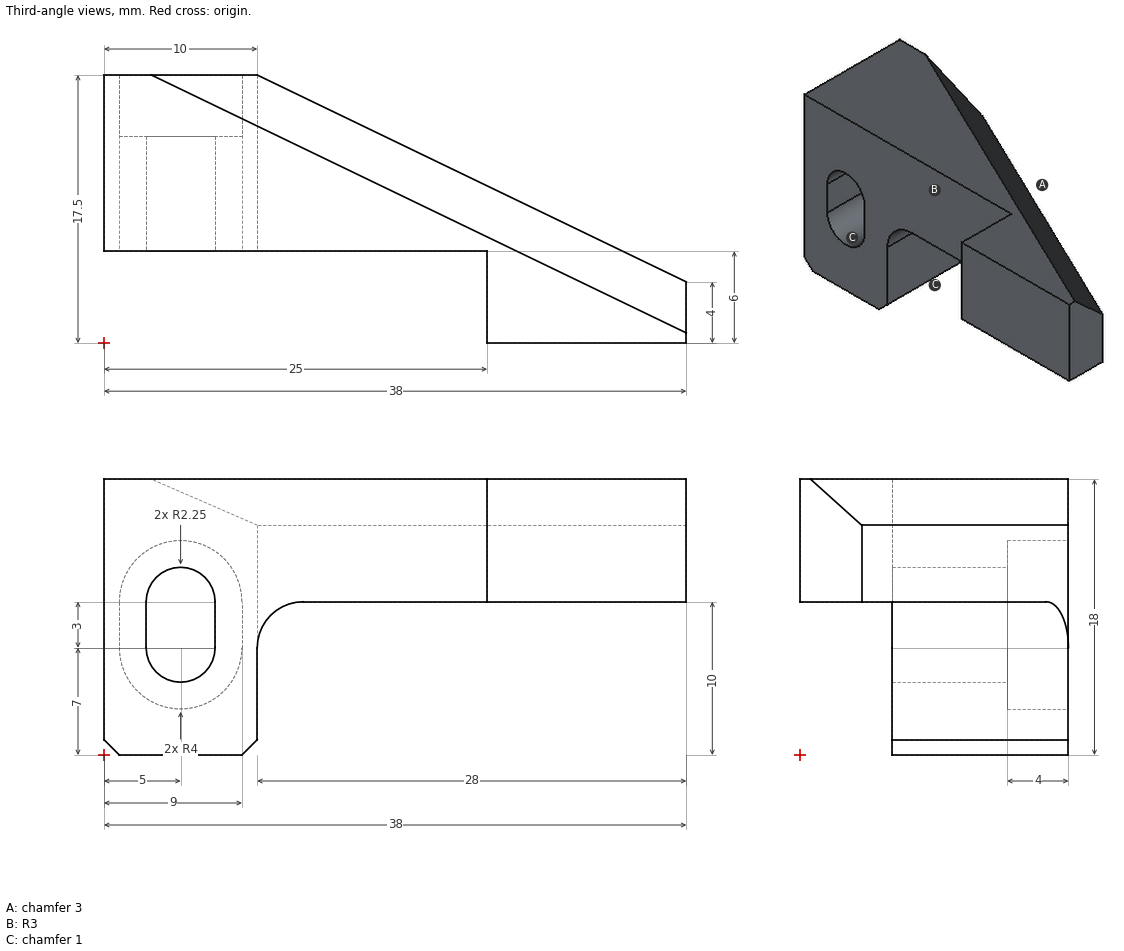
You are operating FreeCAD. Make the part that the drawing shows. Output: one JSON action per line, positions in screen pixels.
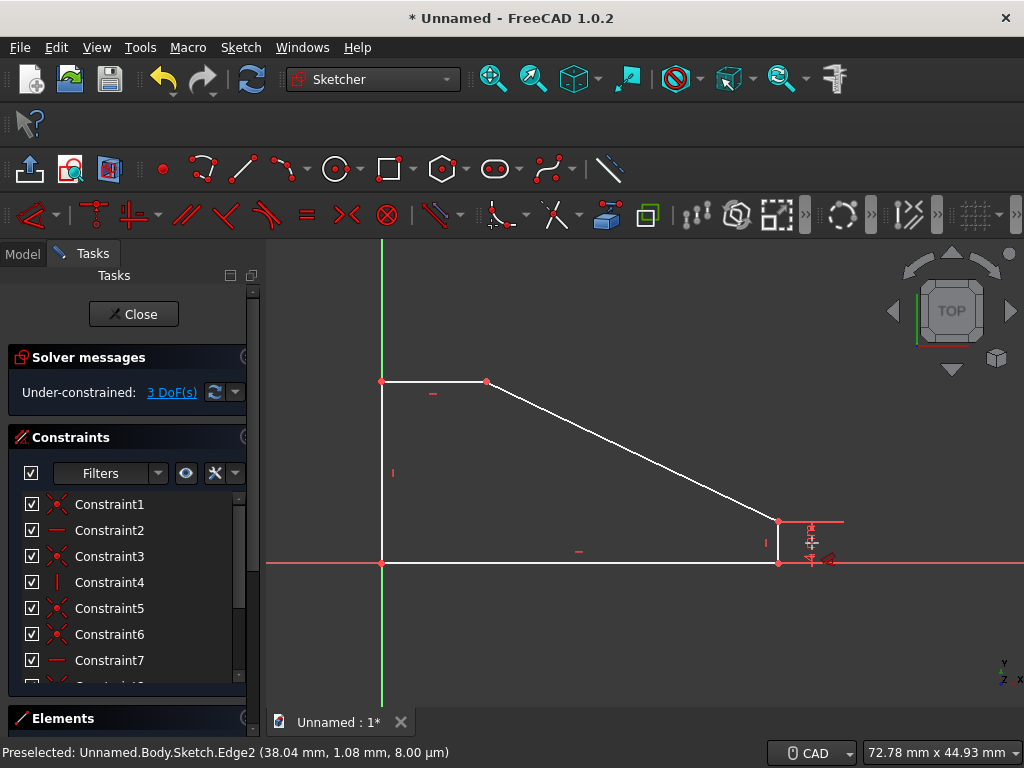
{"action": "left_click", "coordinate": [501, 563]}
{"action": "left_click", "coordinate": [580, 597]}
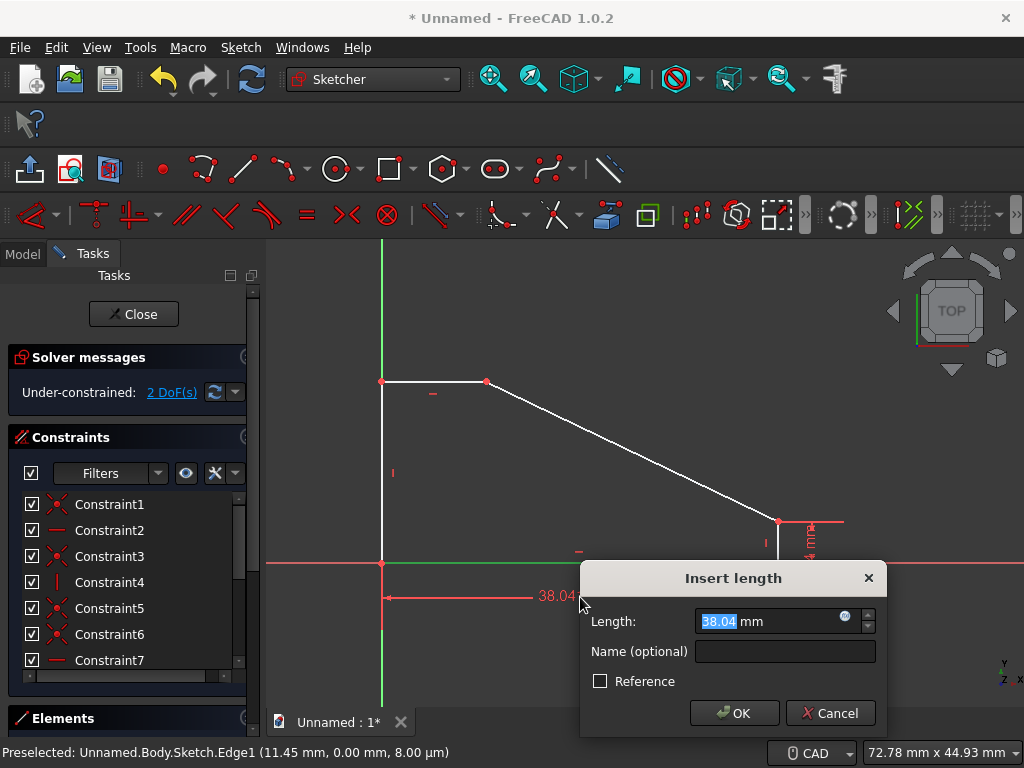
{"action": "type", "text": "38"}
{"action": "key", "text": "Return"}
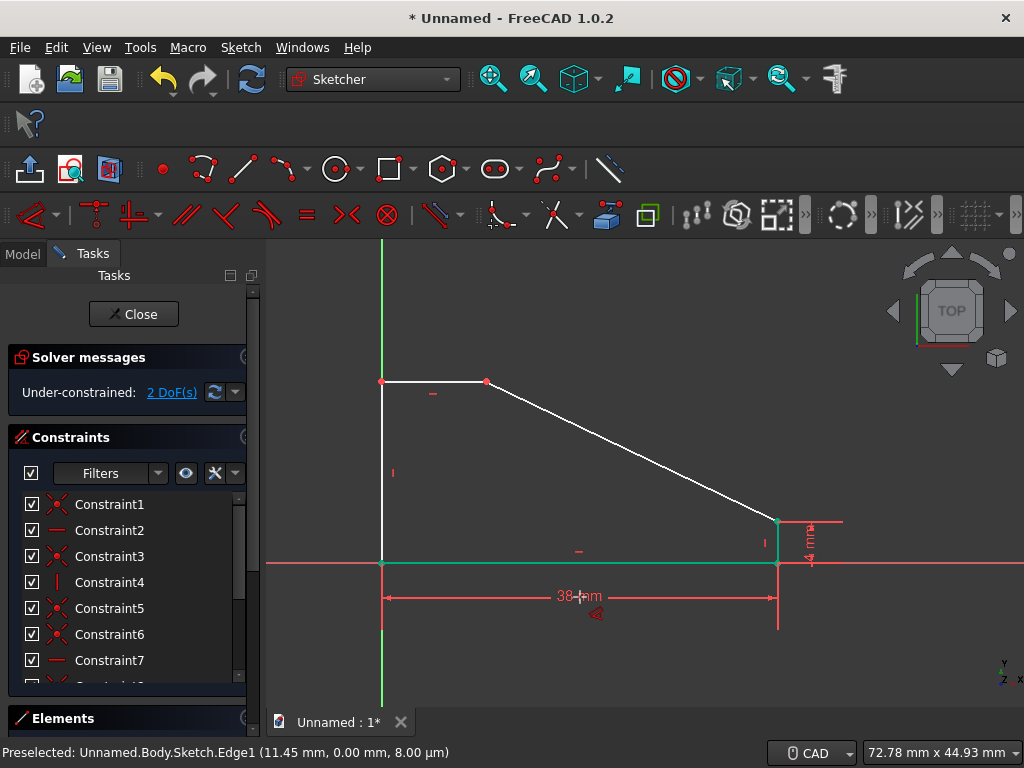
{"action": "left_click", "coordinate": [455, 382]}
{"action": "left_click", "coordinate": [434, 348]}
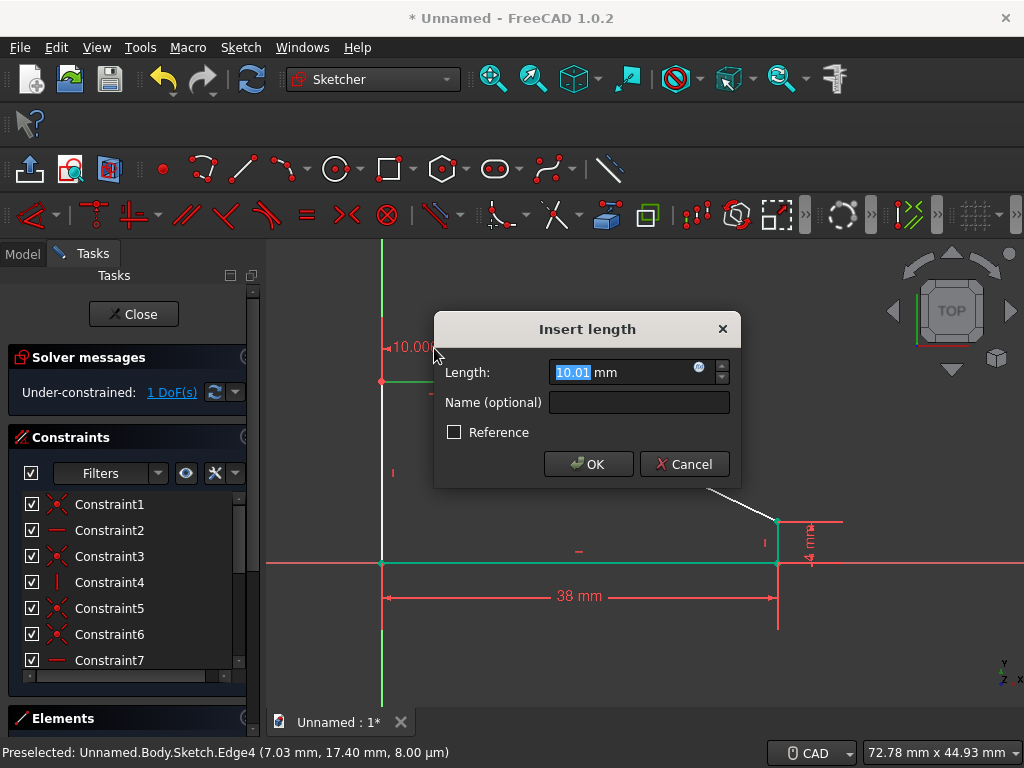
{"action": "type", "text": "10"}
{"action": "key", "text": "Return"}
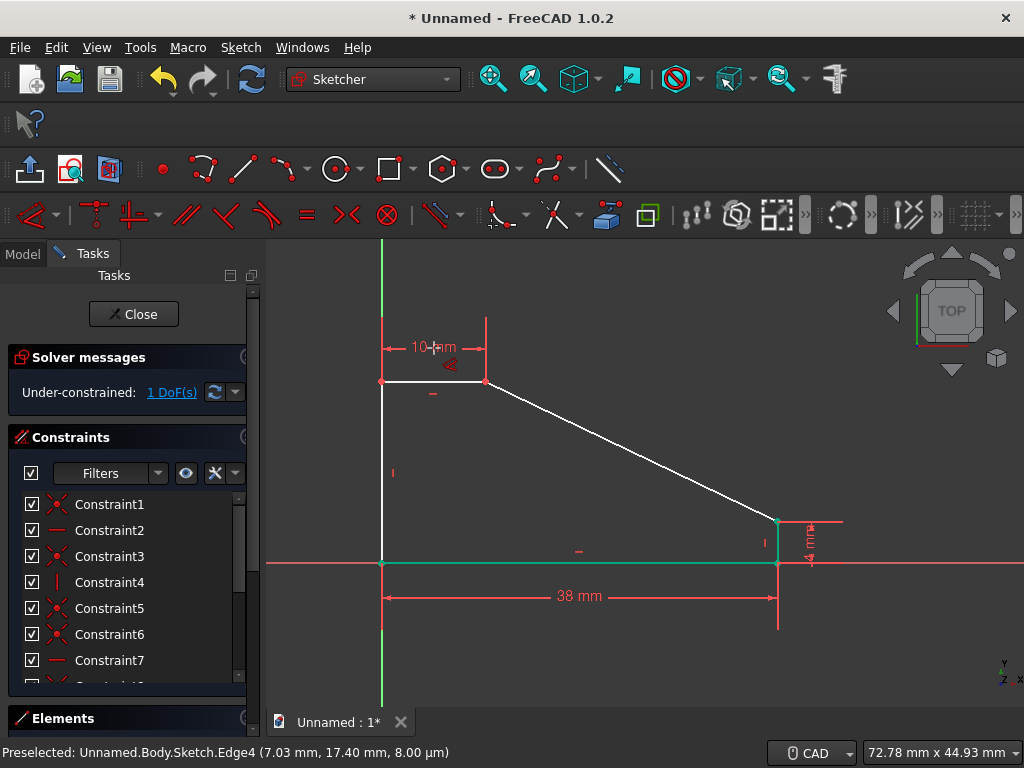
{"action": "left_click", "coordinate": [382, 436]}
{"action": "left_click", "coordinate": [348, 473]}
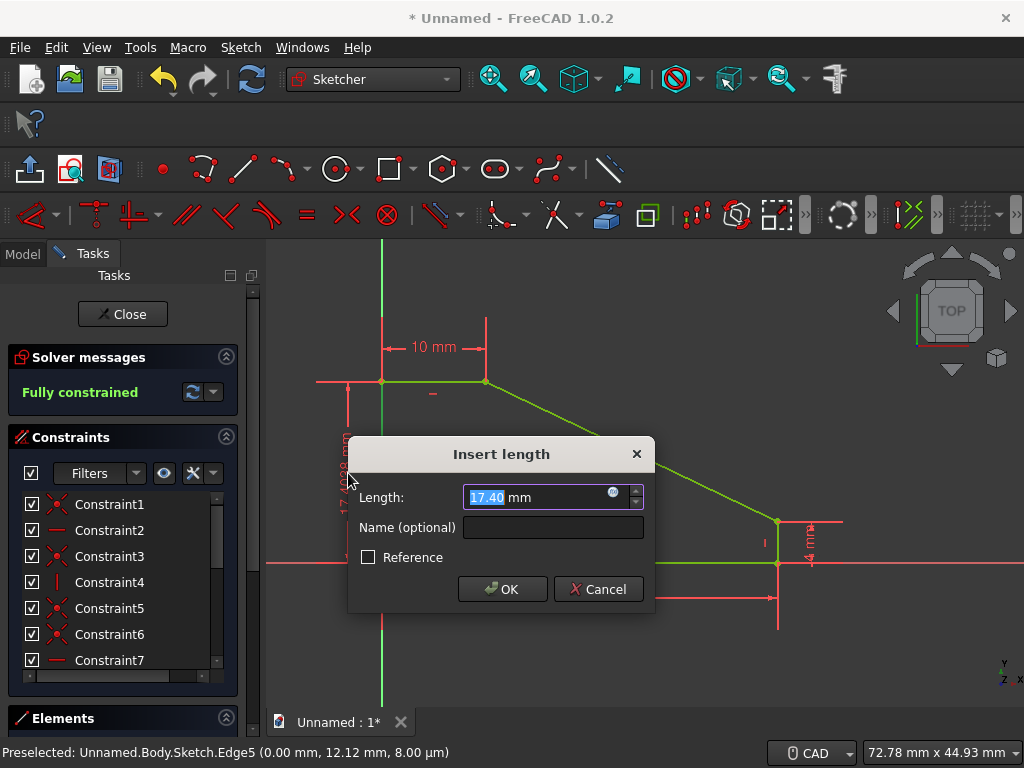
{"action": "type", "text": "17.5"}
{"action": "key", "text": "Return"}
{"action": "key", "text": "Escape"}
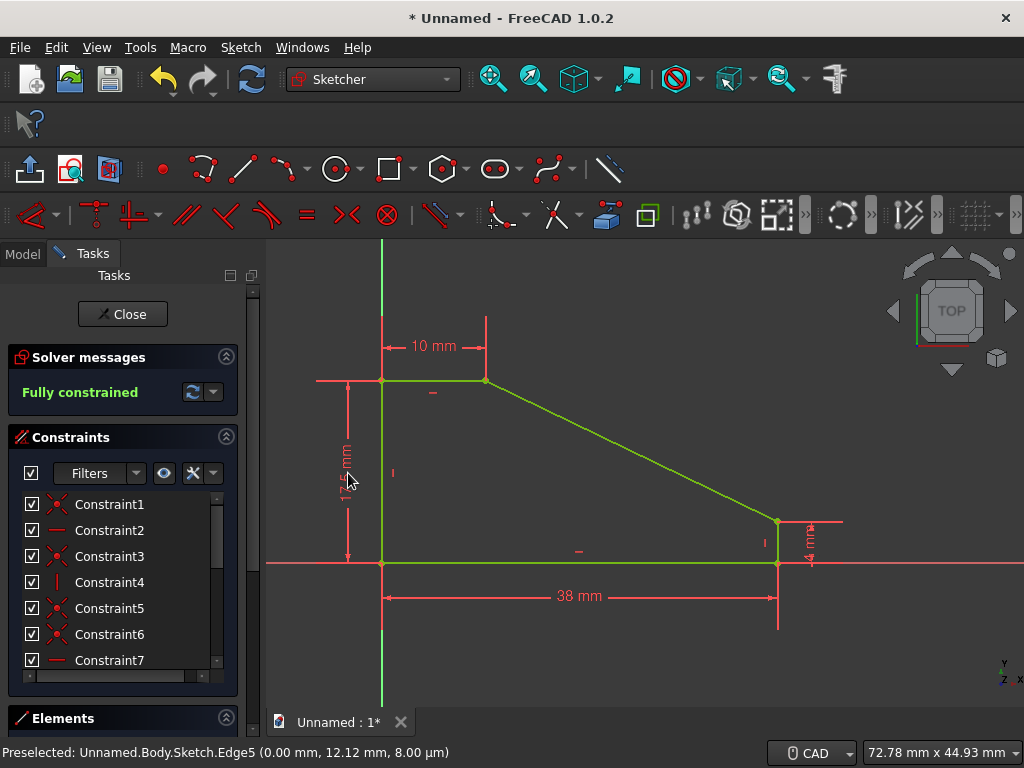
{"action": "left_click", "coordinate": [123, 314]}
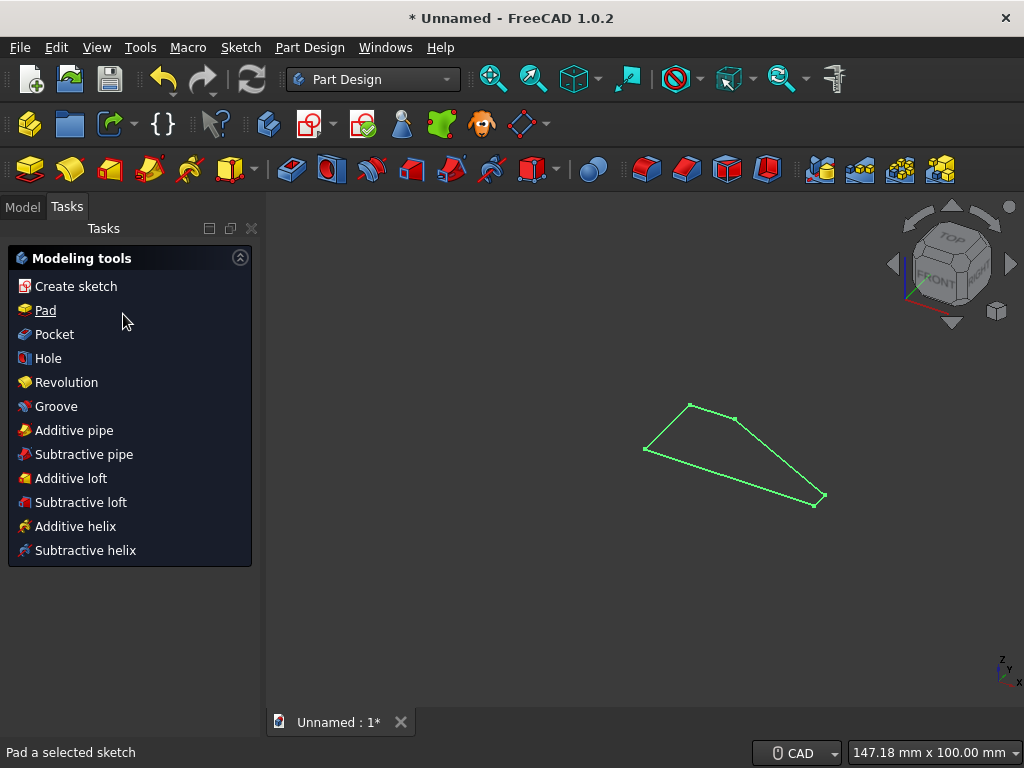
{"action": "left_click", "coordinate": [30, 170]}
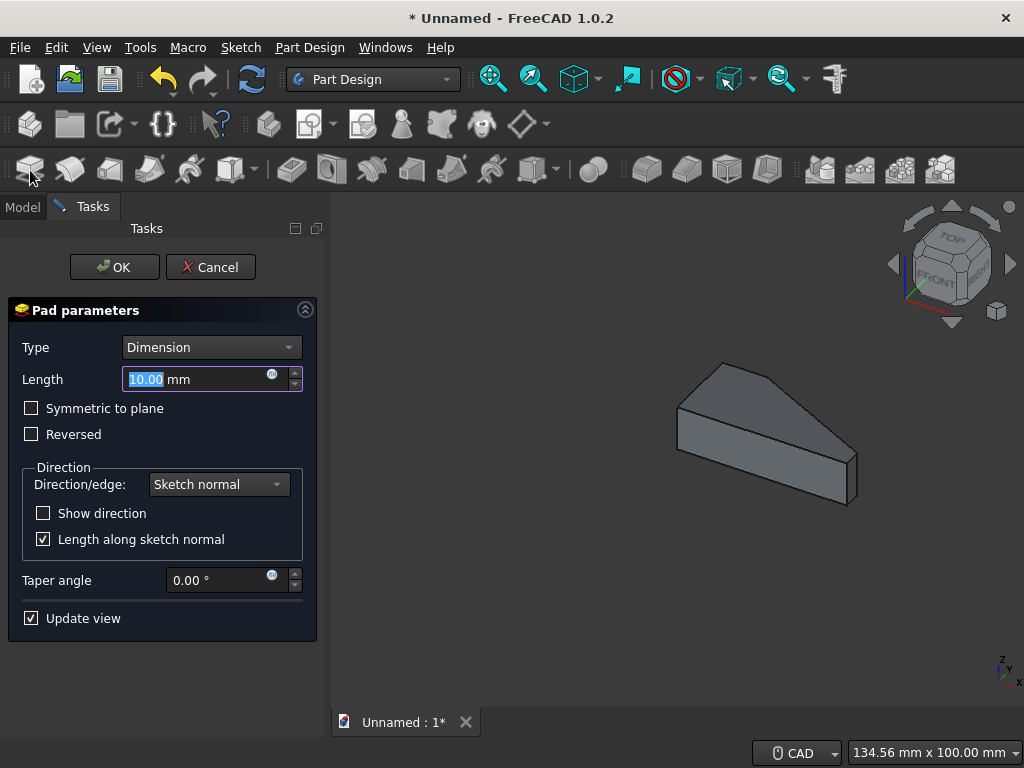
{"action": "type", "text": "18"}
{"action": "key", "text": "Tab"}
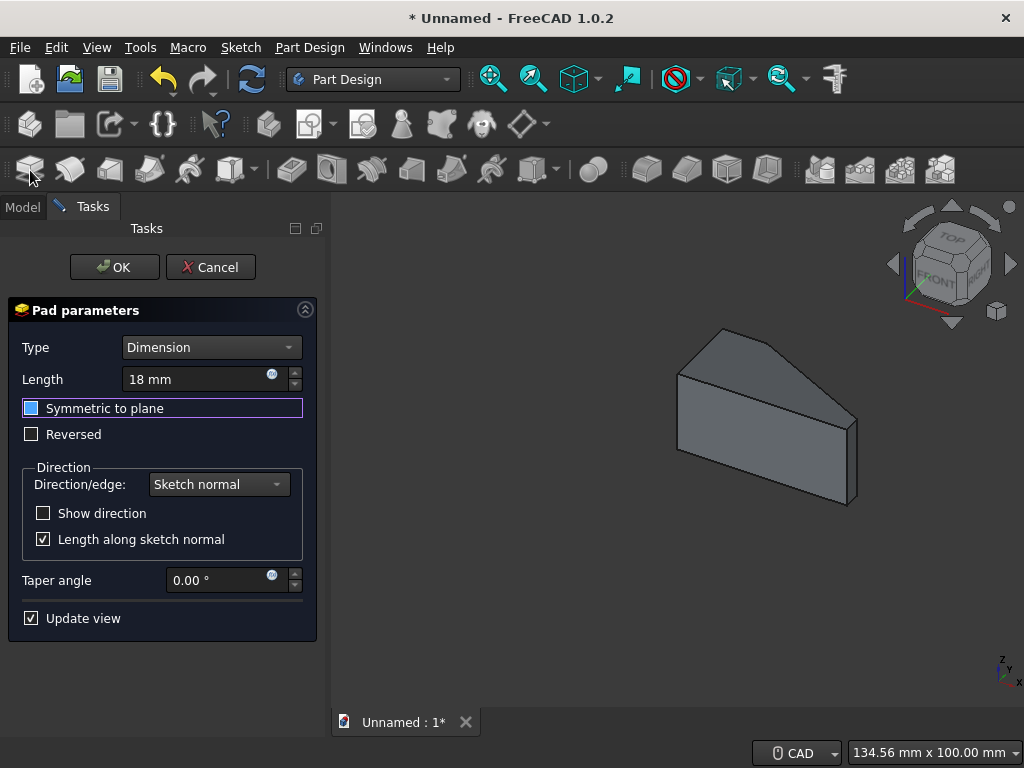
{"action": "left_click", "coordinate": [115, 267]}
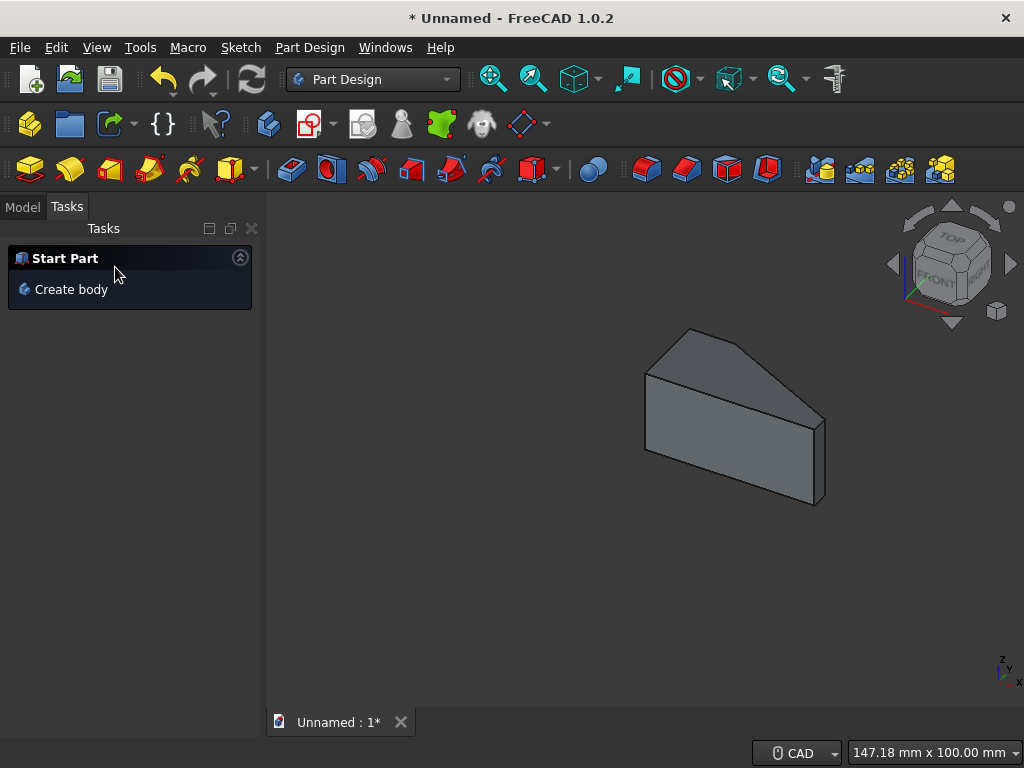
{"action": "left_click", "coordinate": [494, 80]}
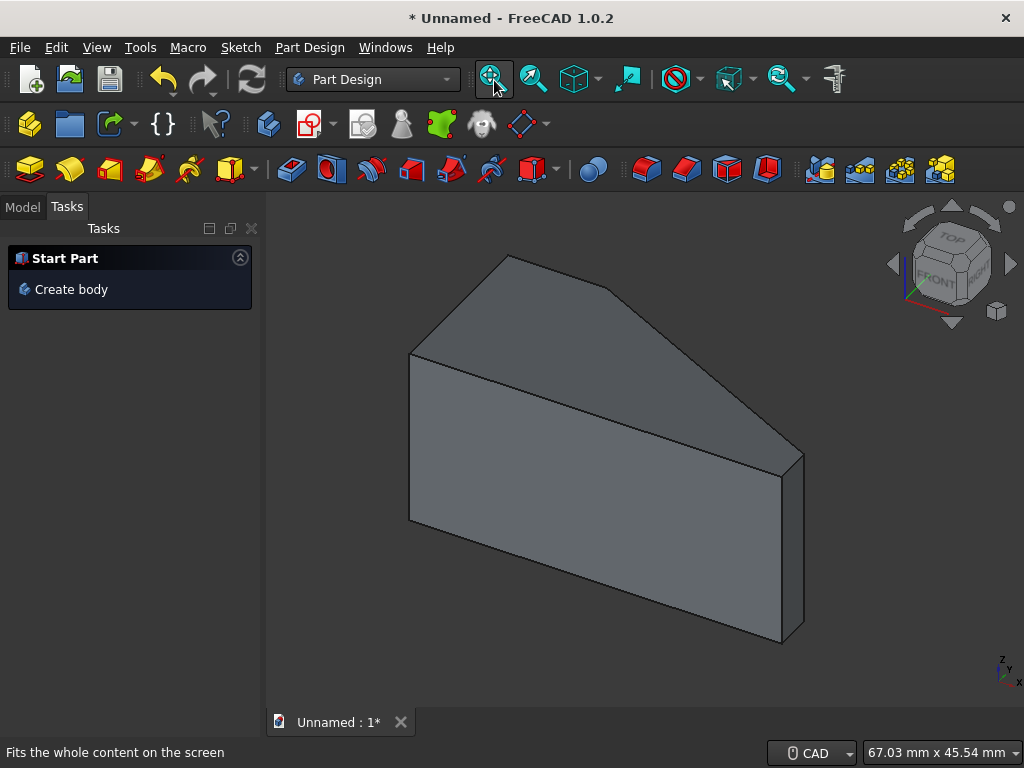
{"action": "key", "text": "0"}